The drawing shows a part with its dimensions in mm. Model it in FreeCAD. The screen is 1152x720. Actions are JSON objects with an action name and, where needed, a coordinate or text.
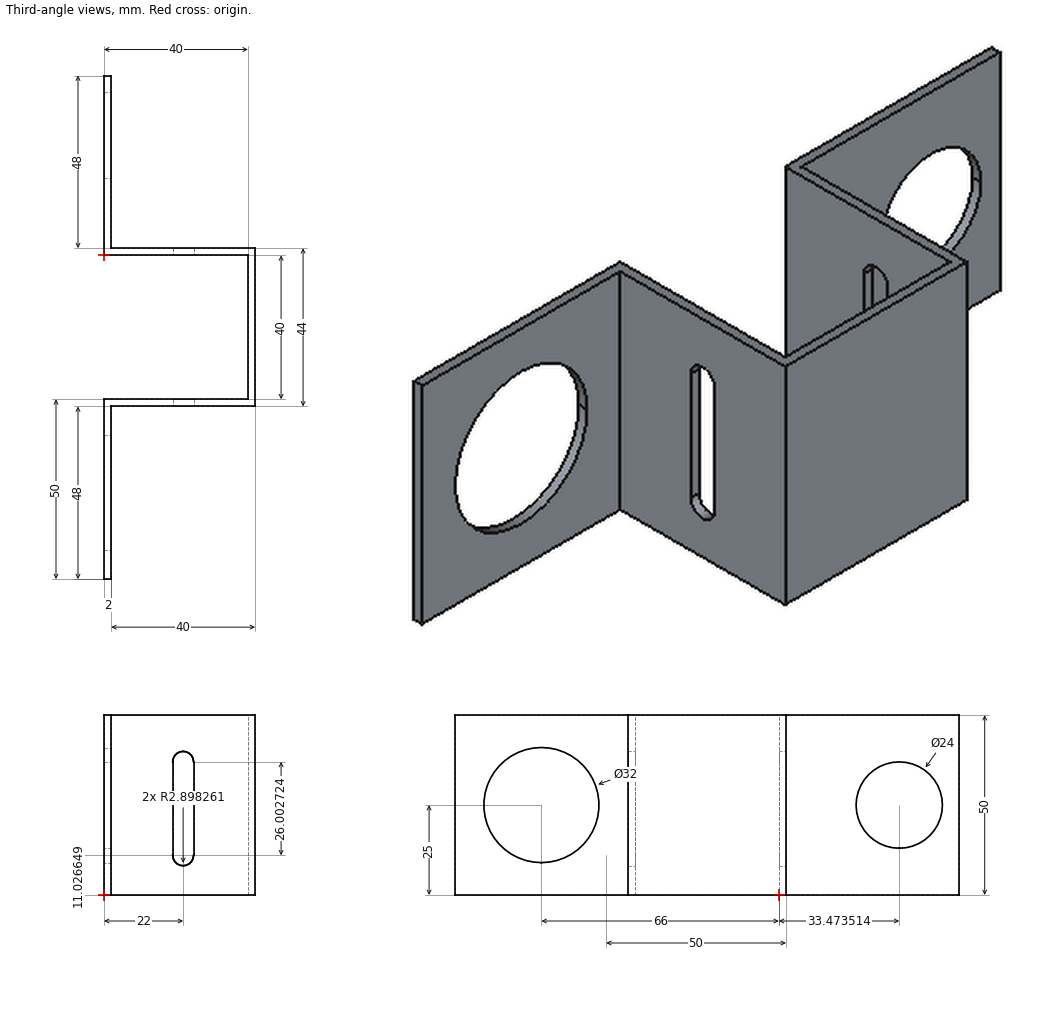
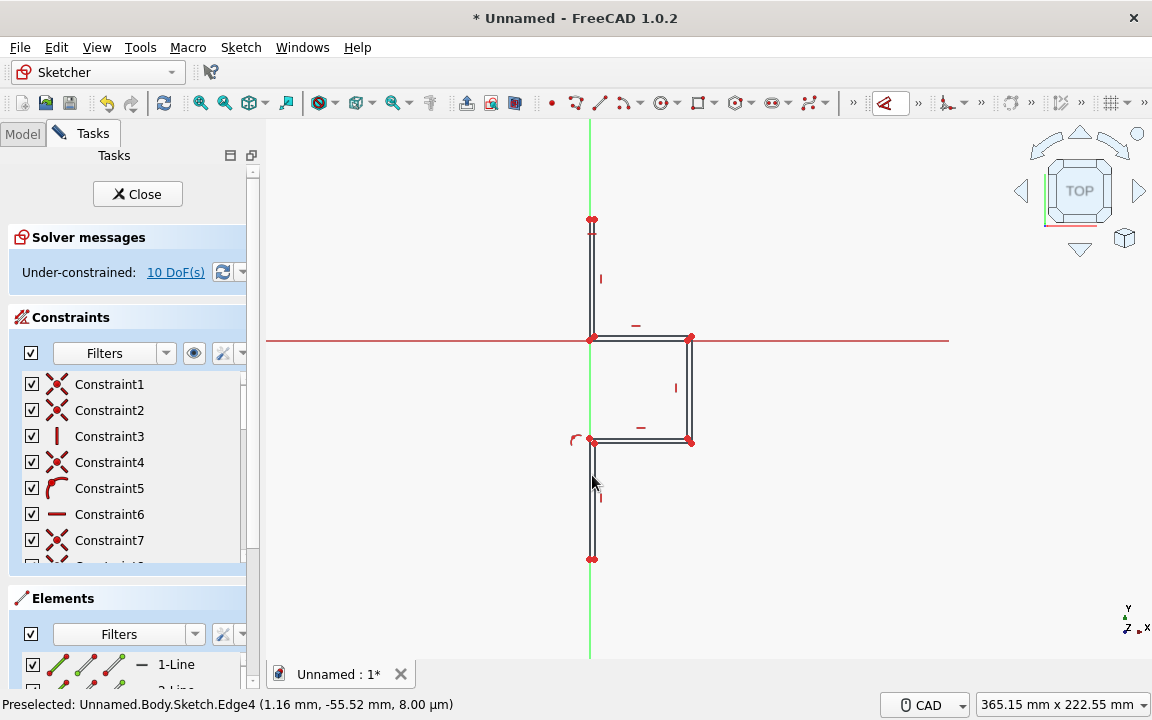
{"action": "scroll", "coordinate": [591, 560], "scroll_direction": "up", "scroll_amount": 12}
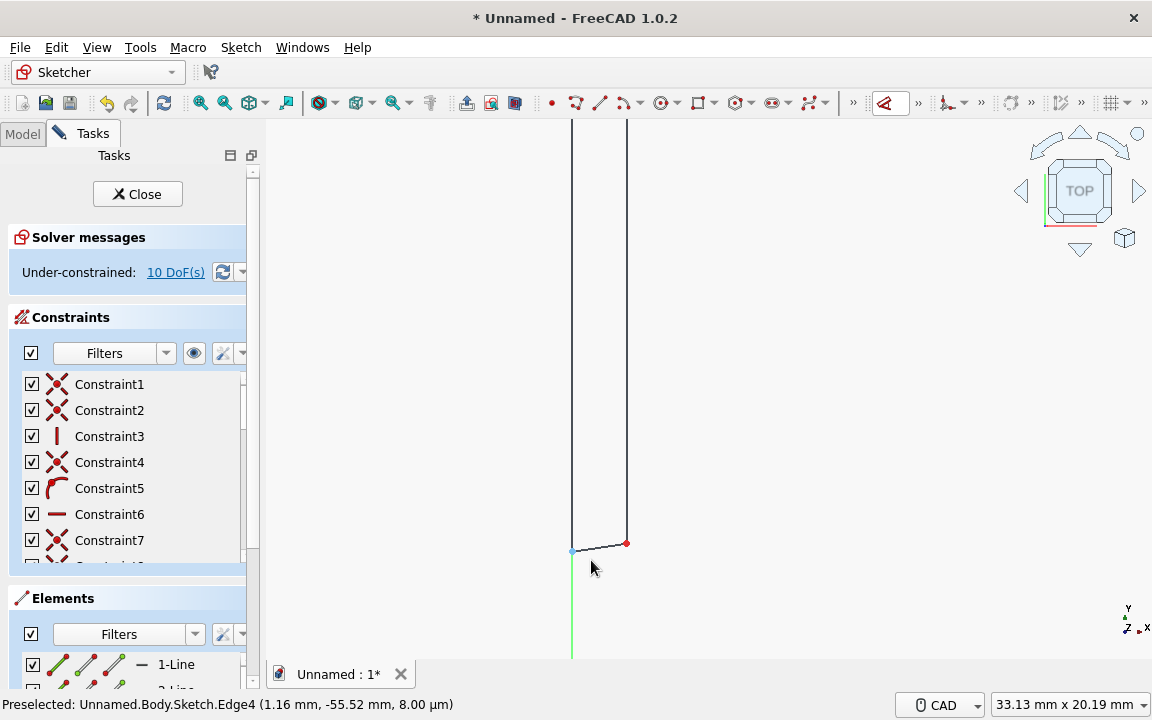
{"action": "left_click", "coordinate": [589, 549]}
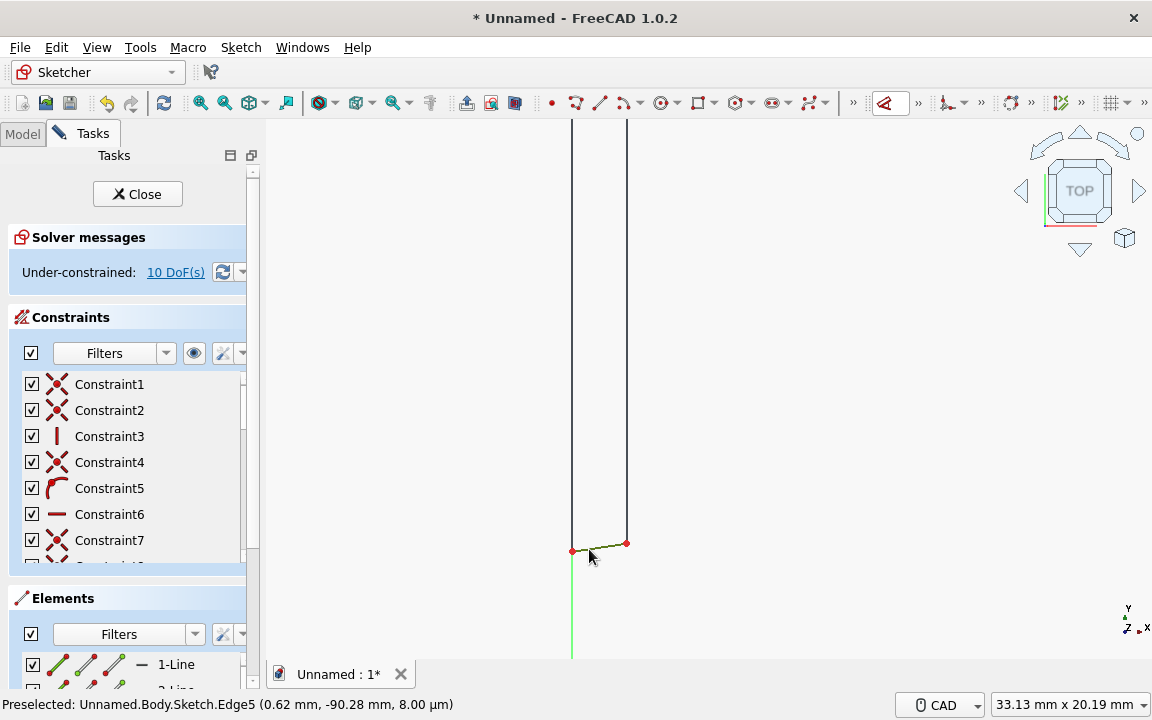
{"action": "key", "text": "h"}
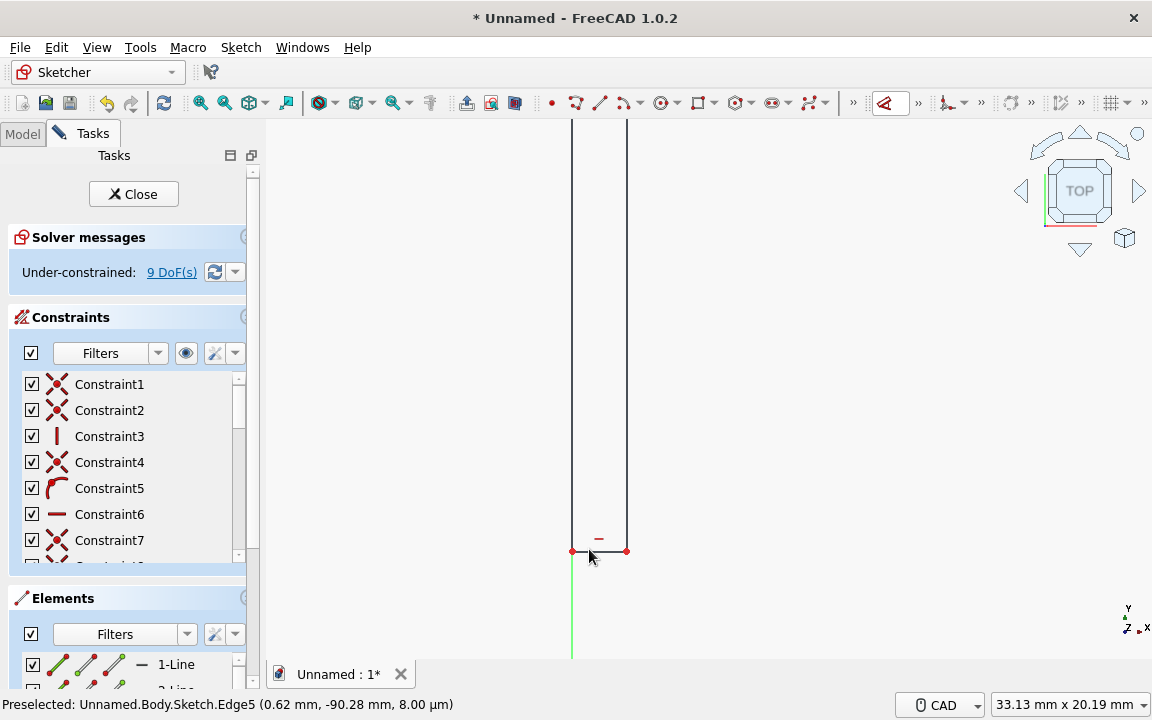
{"action": "left_click", "coordinate": [884, 104]}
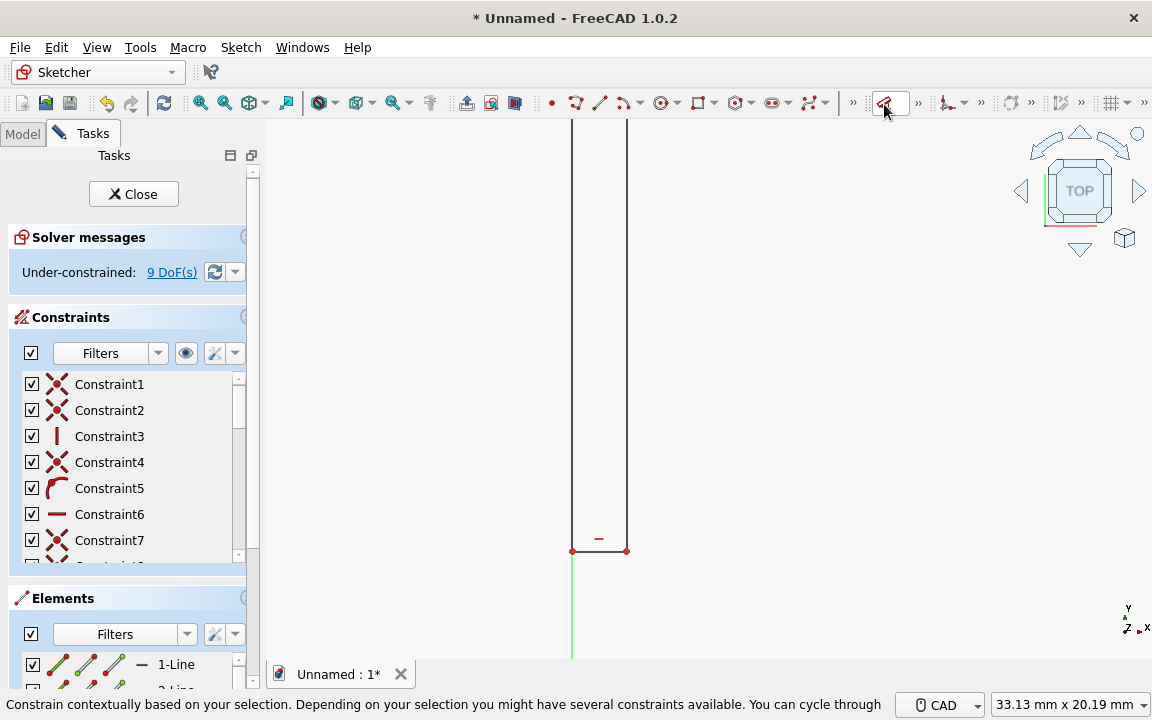
{"action": "left_click", "coordinate": [589, 552]}
{"action": "left_click", "coordinate": [599, 586]}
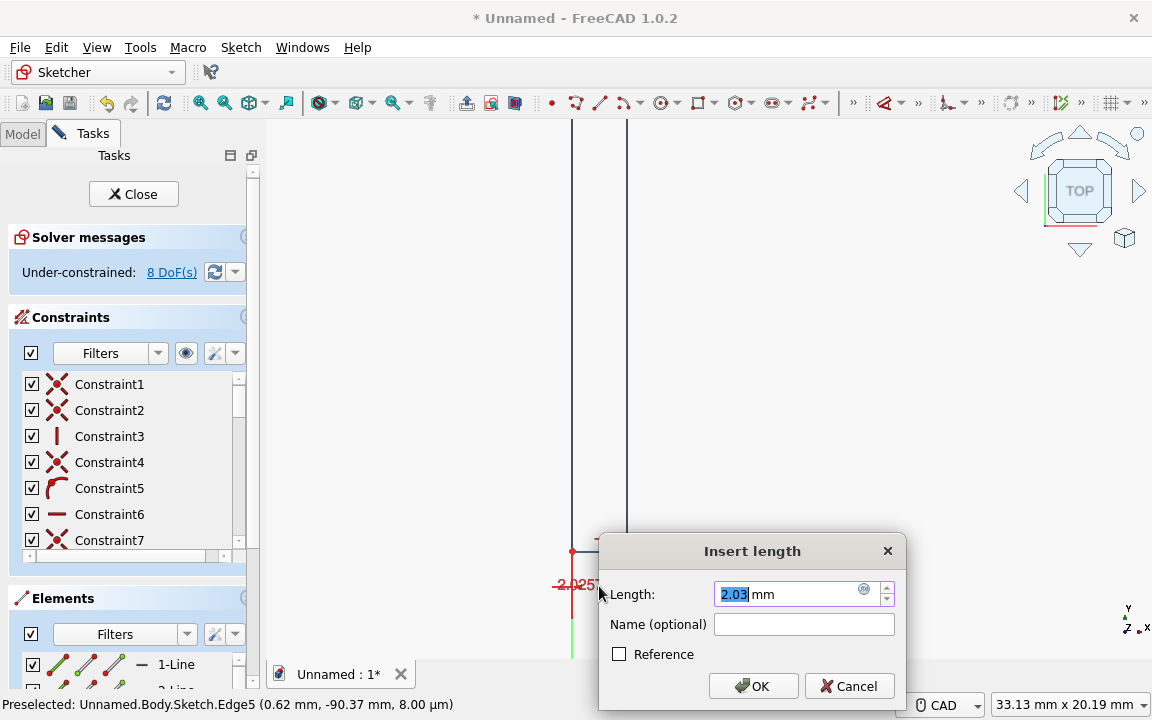
{"action": "type", "text": "2"}
{"action": "key", "text": "Return"}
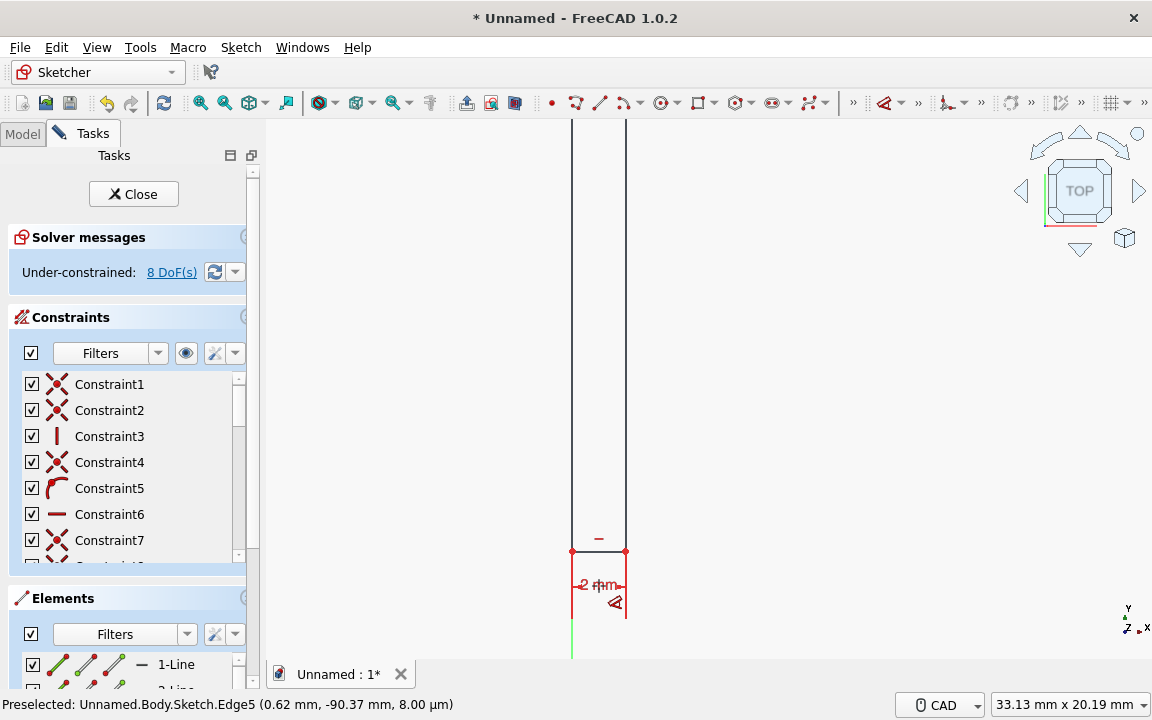
{"action": "scroll", "coordinate": [591, 561], "scroll_direction": "down", "scroll_amount": 12}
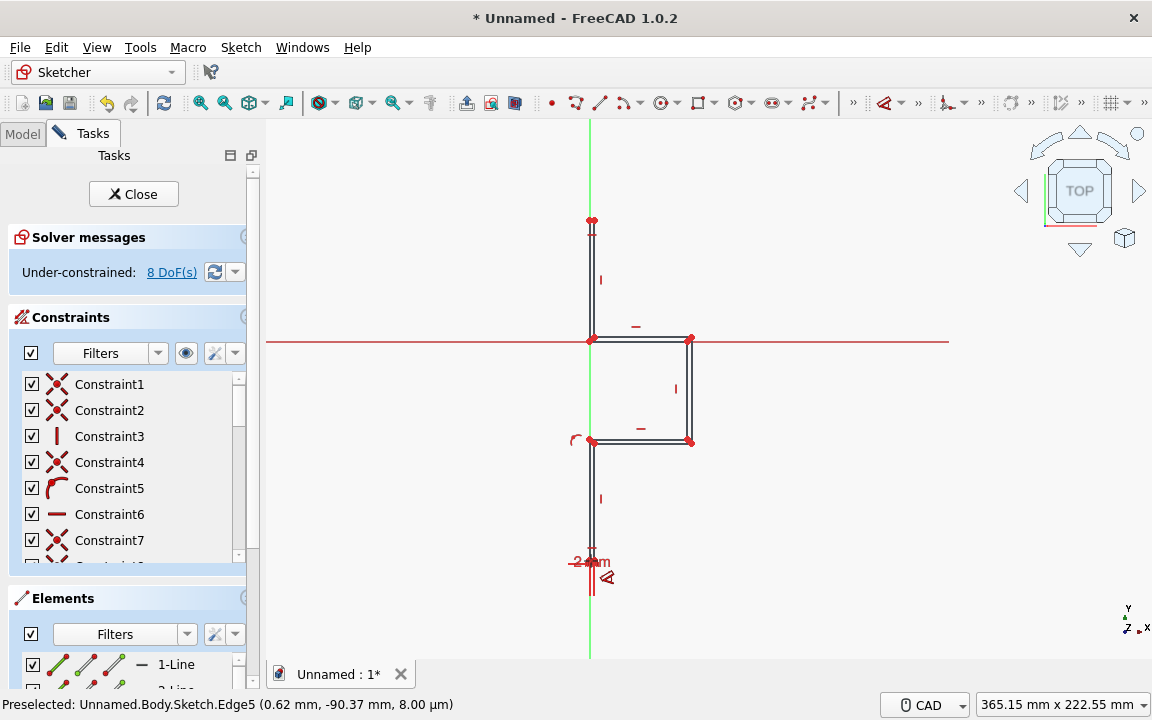
{"action": "scroll", "coordinate": [593, 221], "scroll_direction": "up", "scroll_amount": 12}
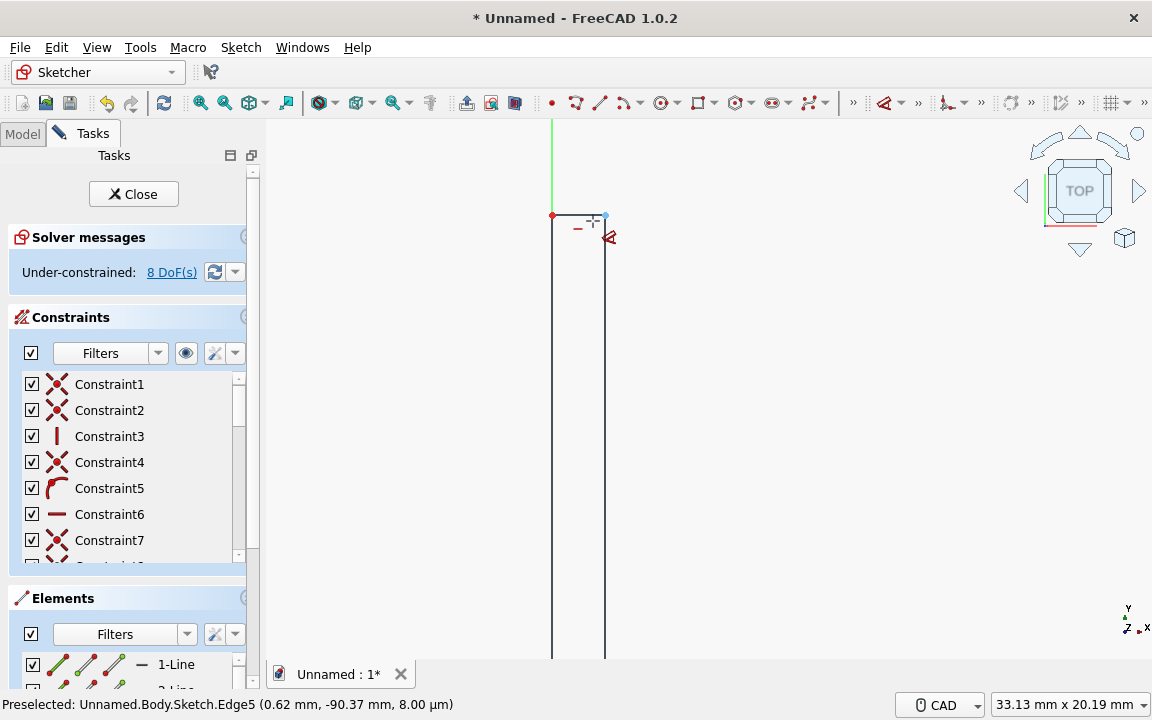
{"action": "left_click", "coordinate": [589, 215]}
{"action": "left_click", "coordinate": [579, 181]}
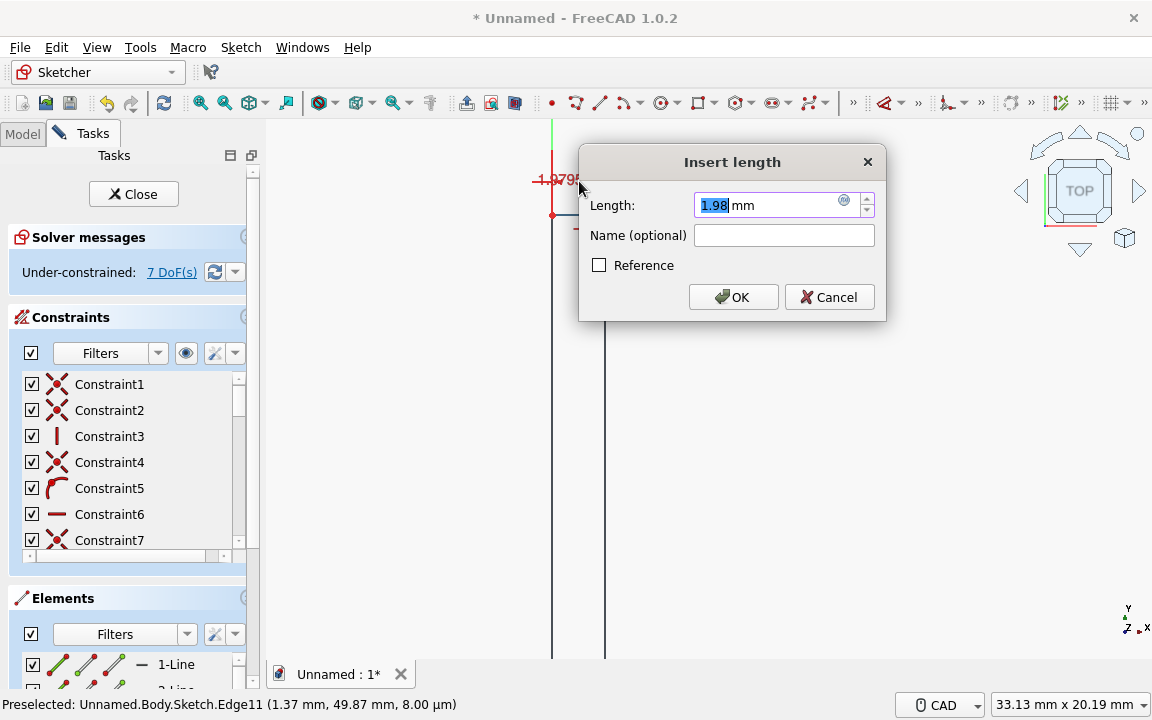
{"action": "type", "text": "2"}
{"action": "key", "text": "Return"}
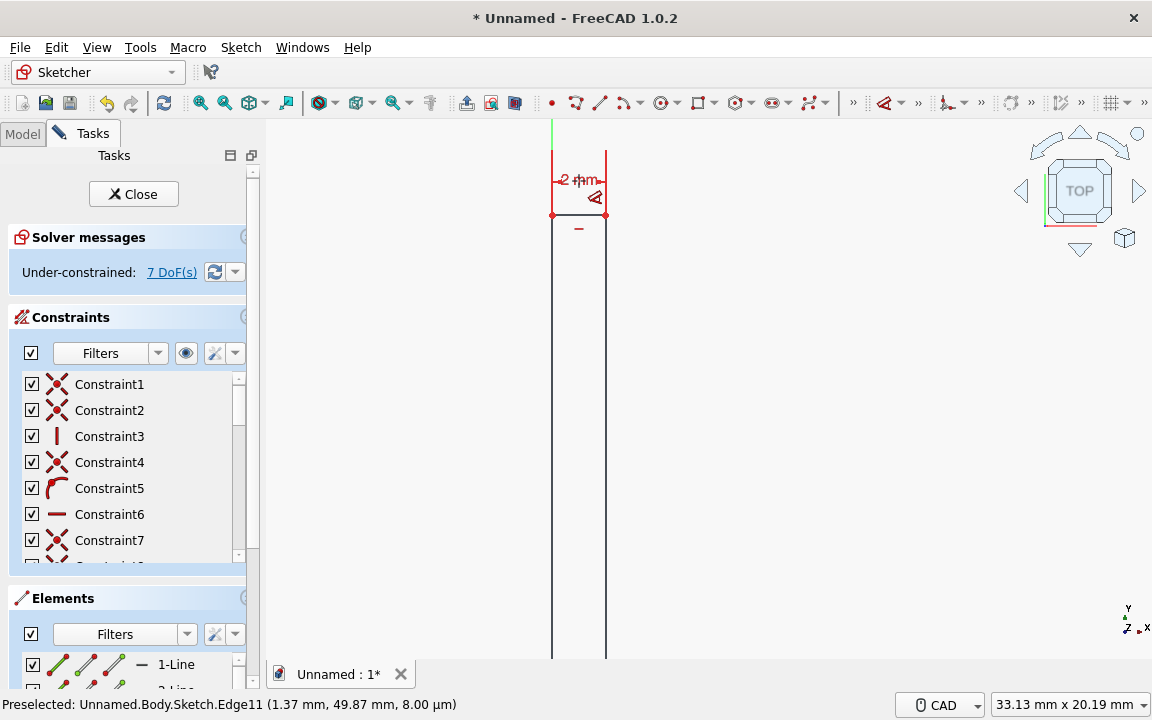
{"action": "scroll", "coordinate": [593, 220], "scroll_direction": "down", "scroll_amount": 12}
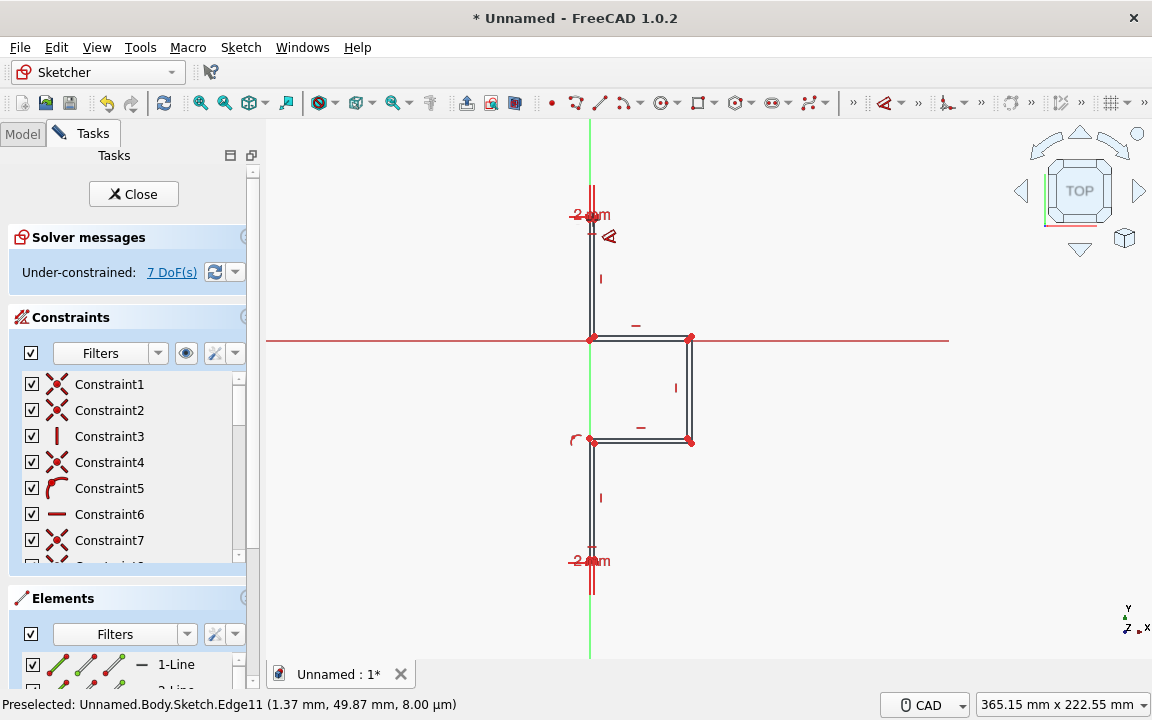
{"action": "scroll", "coordinate": [619, 341], "scroll_direction": "up", "scroll_amount": 6}